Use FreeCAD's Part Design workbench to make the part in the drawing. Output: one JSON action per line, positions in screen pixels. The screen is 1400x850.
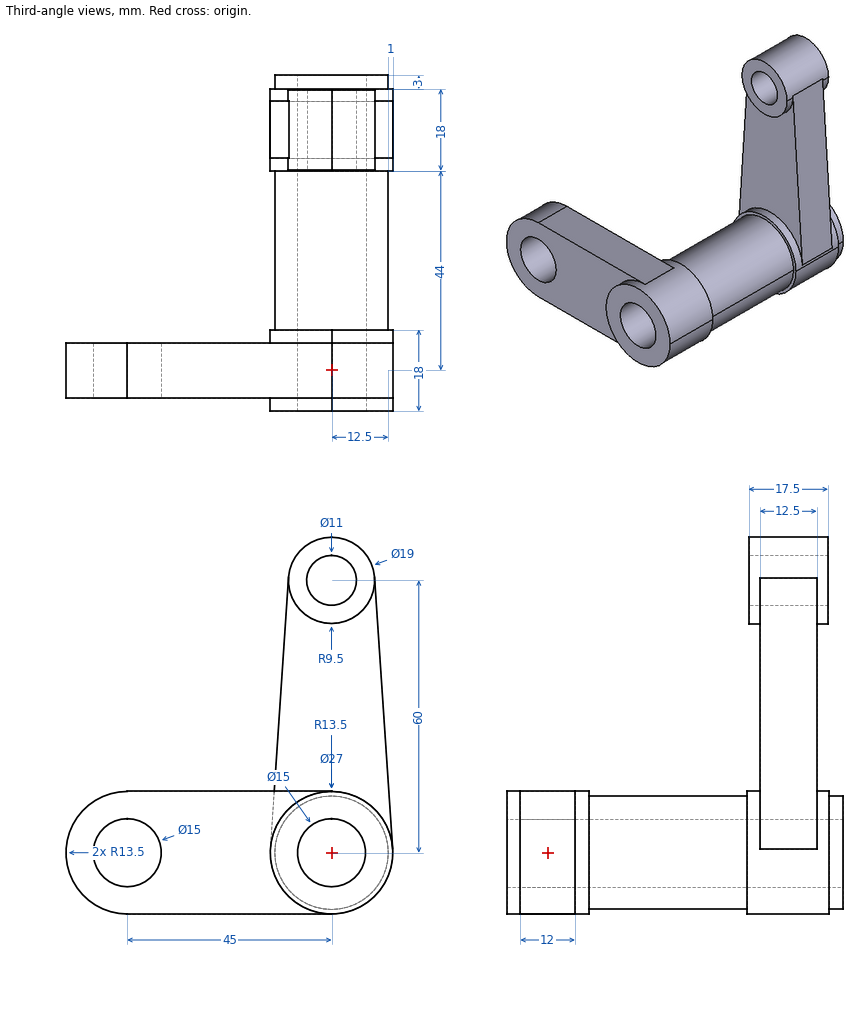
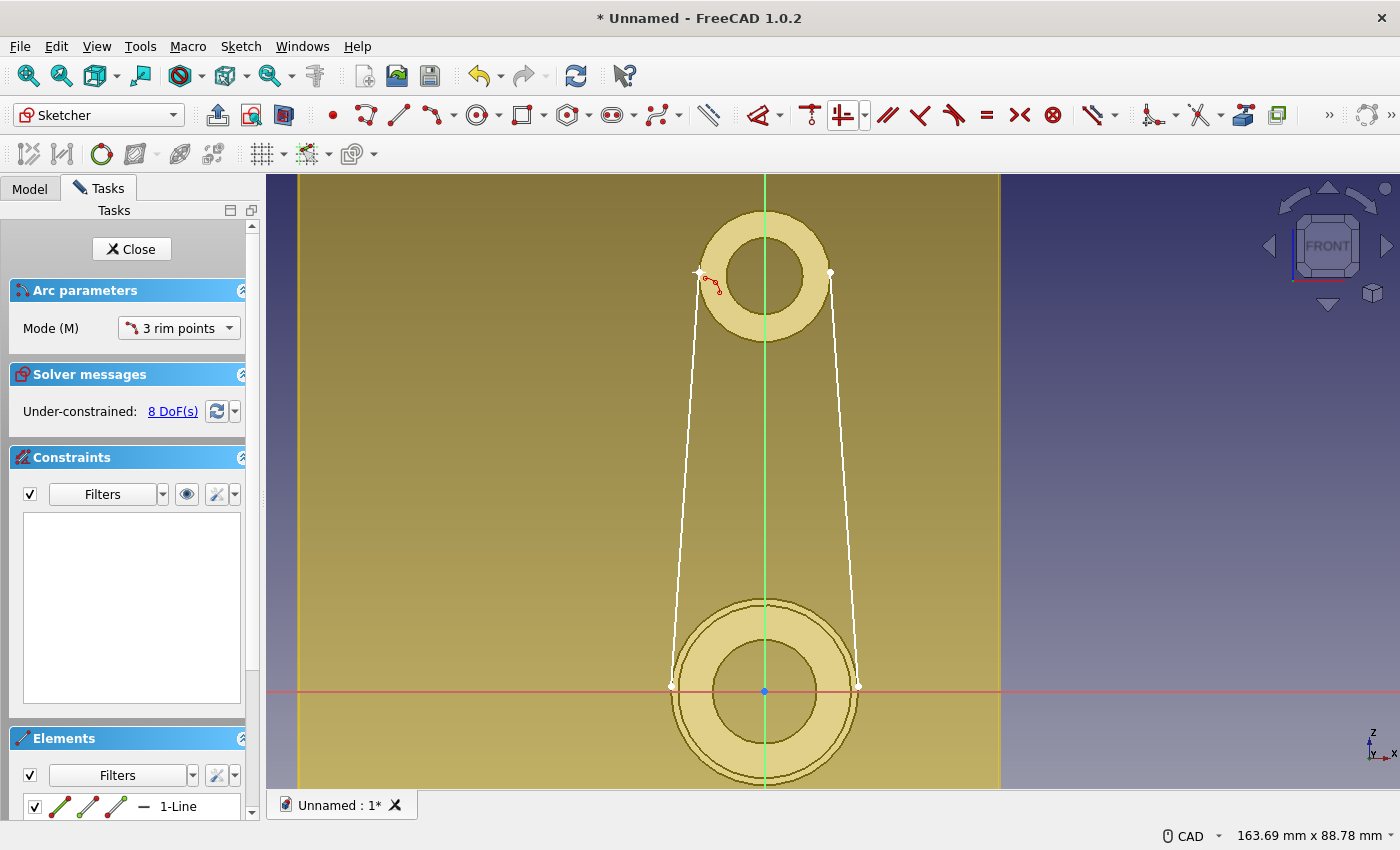
{"action": "scroll", "coordinate": [858, 686], "scroll_direction": "up", "scroll_amount": 5}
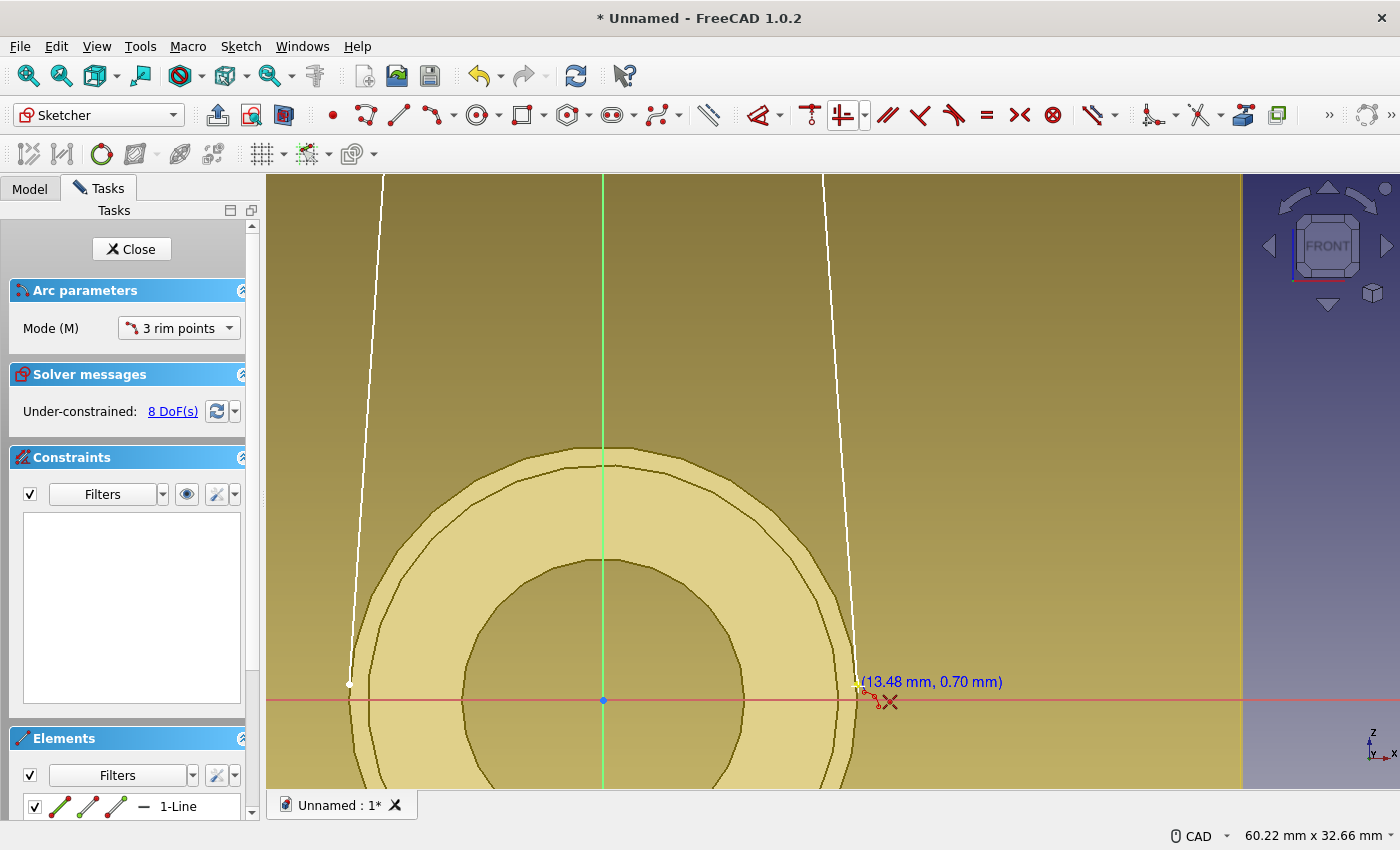
{"action": "left_click", "coordinate": [857, 685]}
{"action": "left_click", "coordinate": [349, 685]}
{"action": "left_click", "coordinate": [679, 458]}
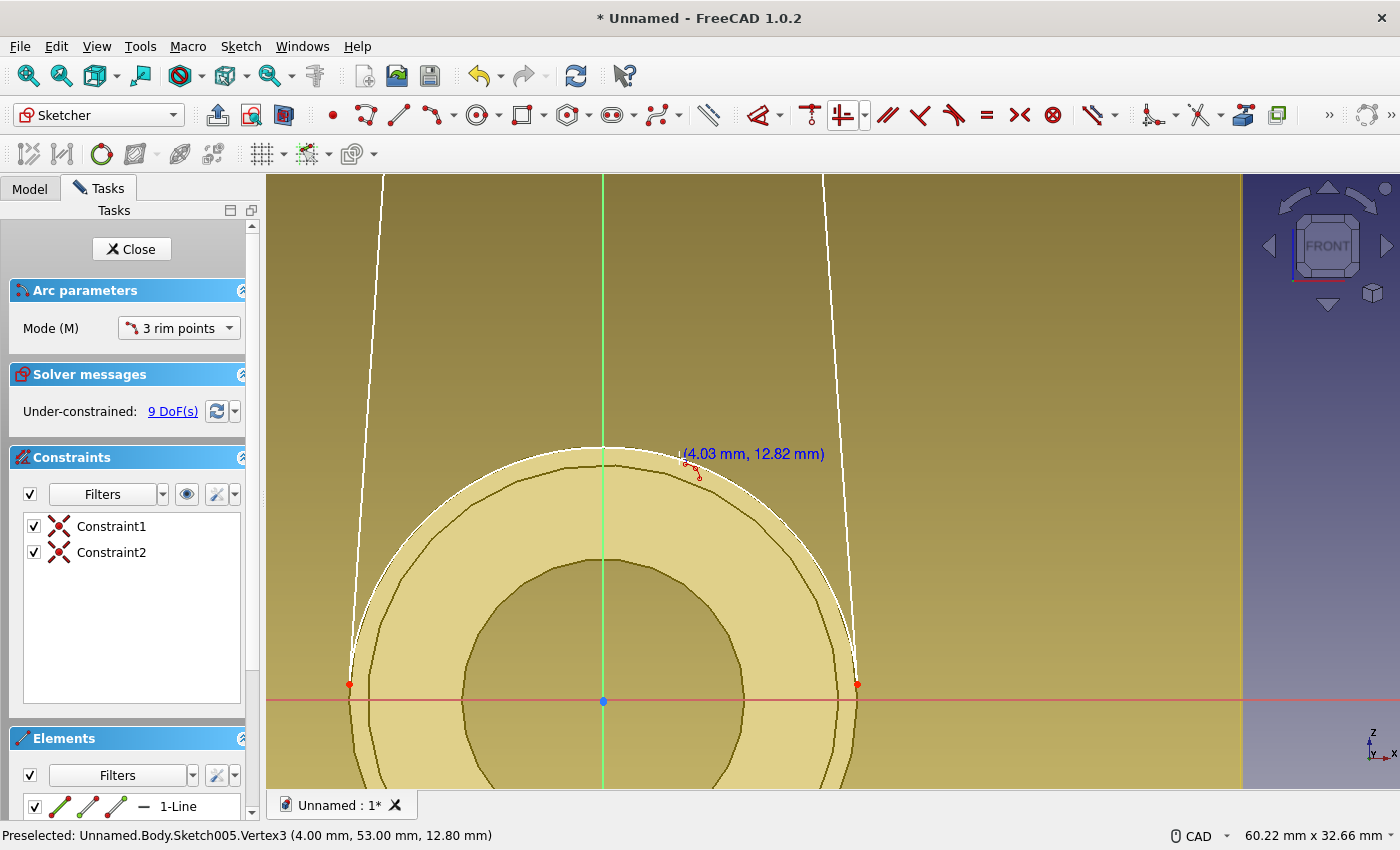
{"action": "scroll", "coordinate": [858, 686], "scroll_direction": "down", "scroll_amount": 5}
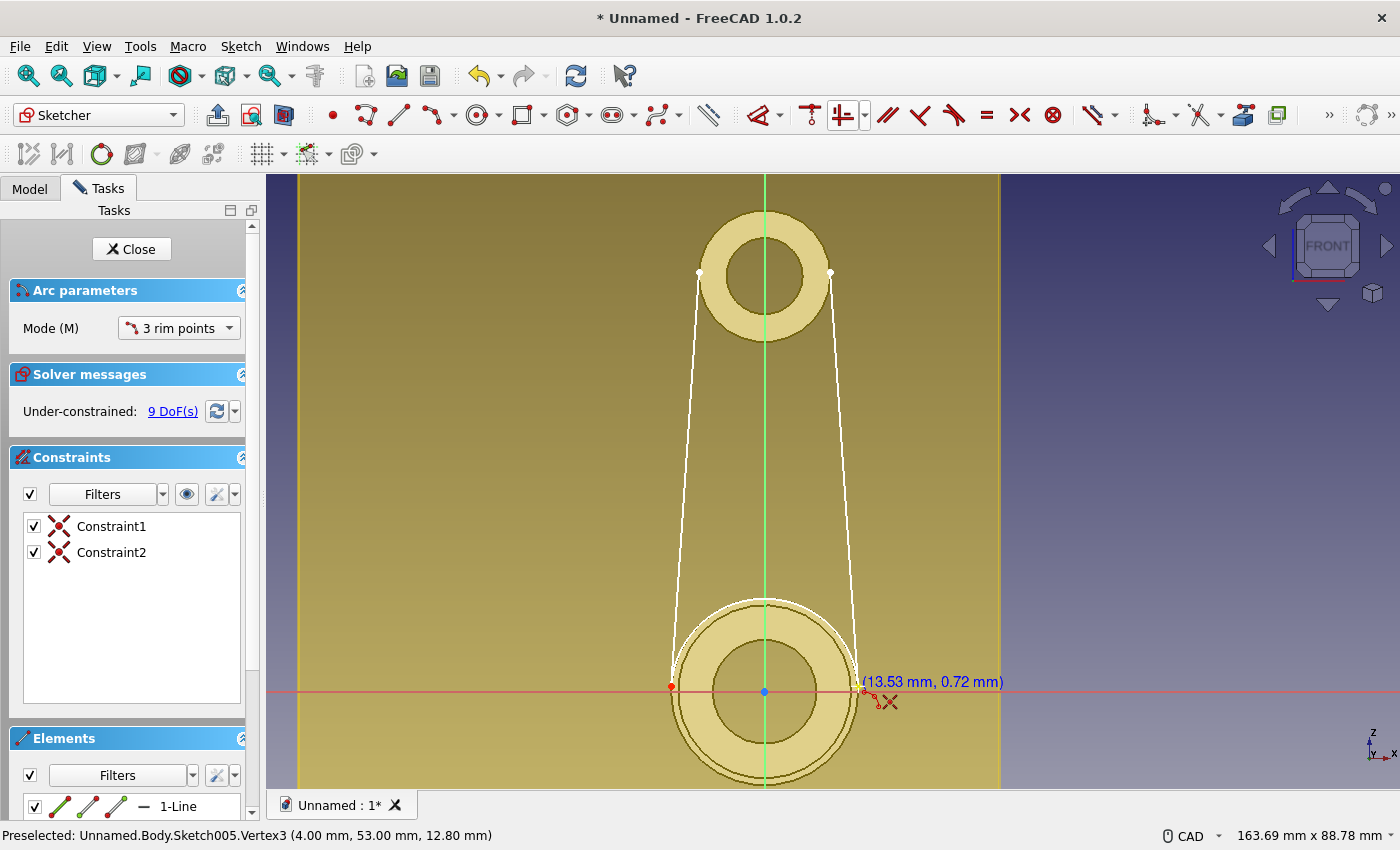
{"action": "left_click", "coordinate": [699, 273]}
{"action": "left_click", "coordinate": [830, 273]}
{"action": "left_click", "coordinate": [743, 339]}
{"action": "key", "text": "Escape"}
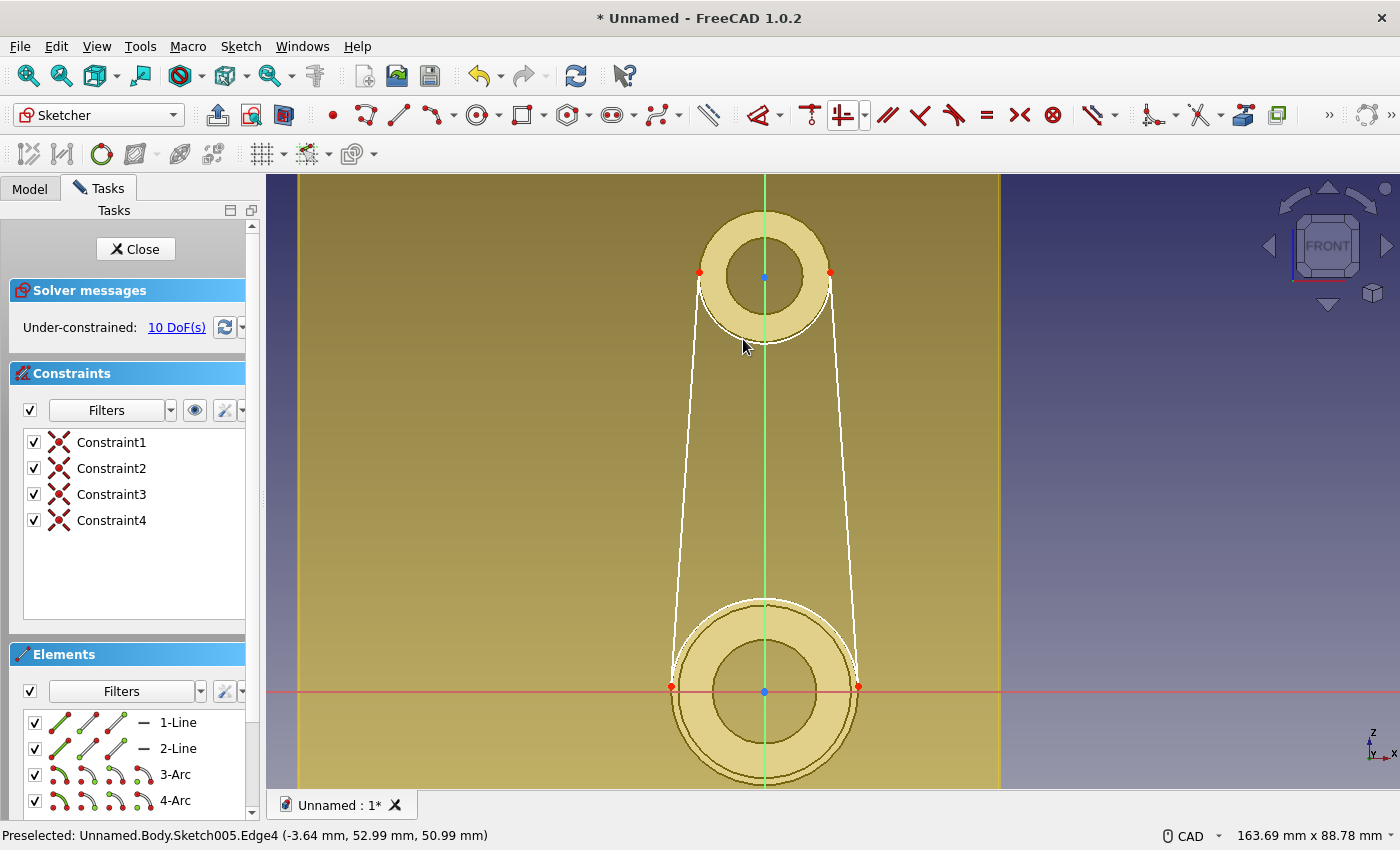
{"action": "left_click", "coordinate": [838, 397]}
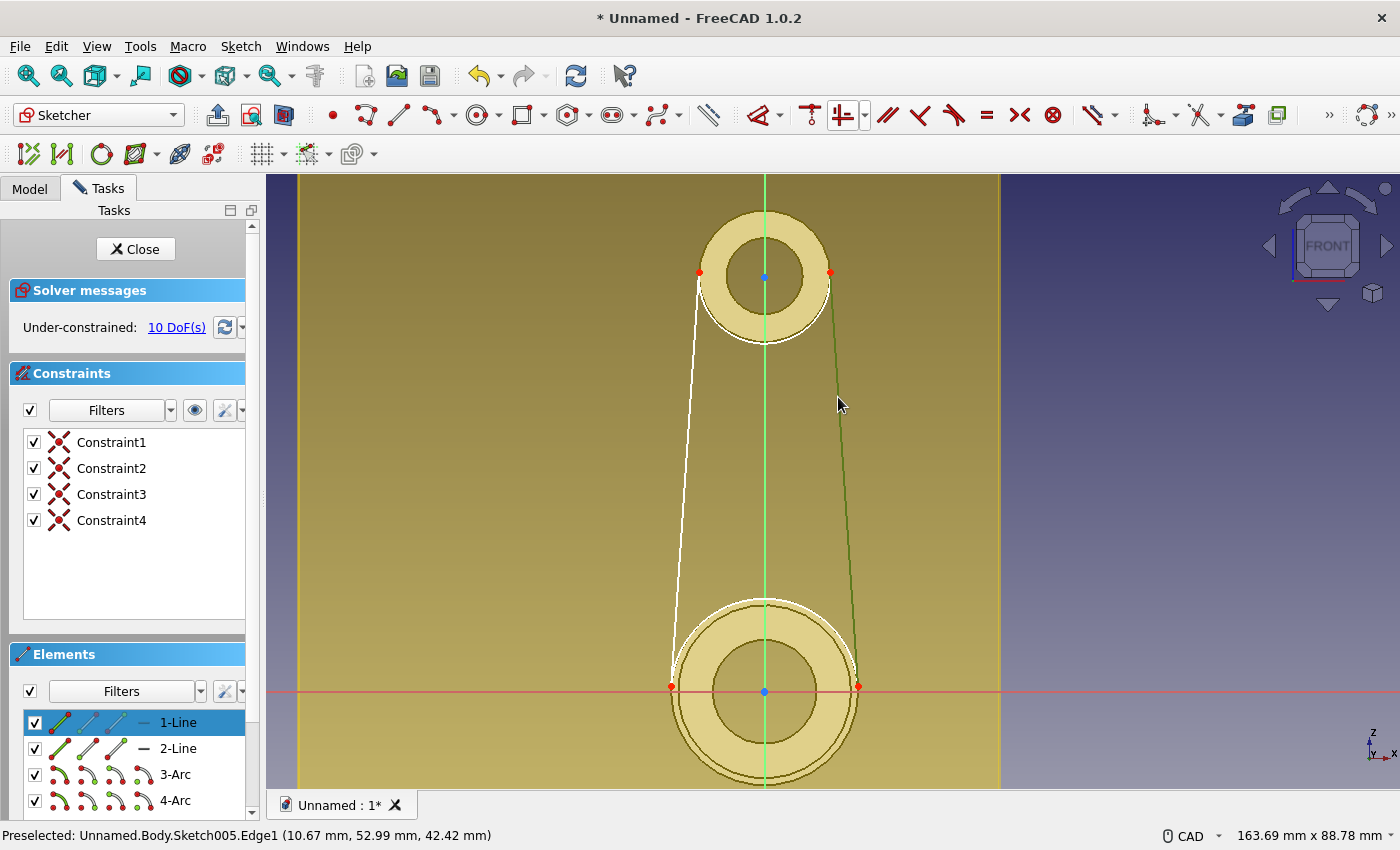
{"action": "left_click", "coordinate": [818, 615]}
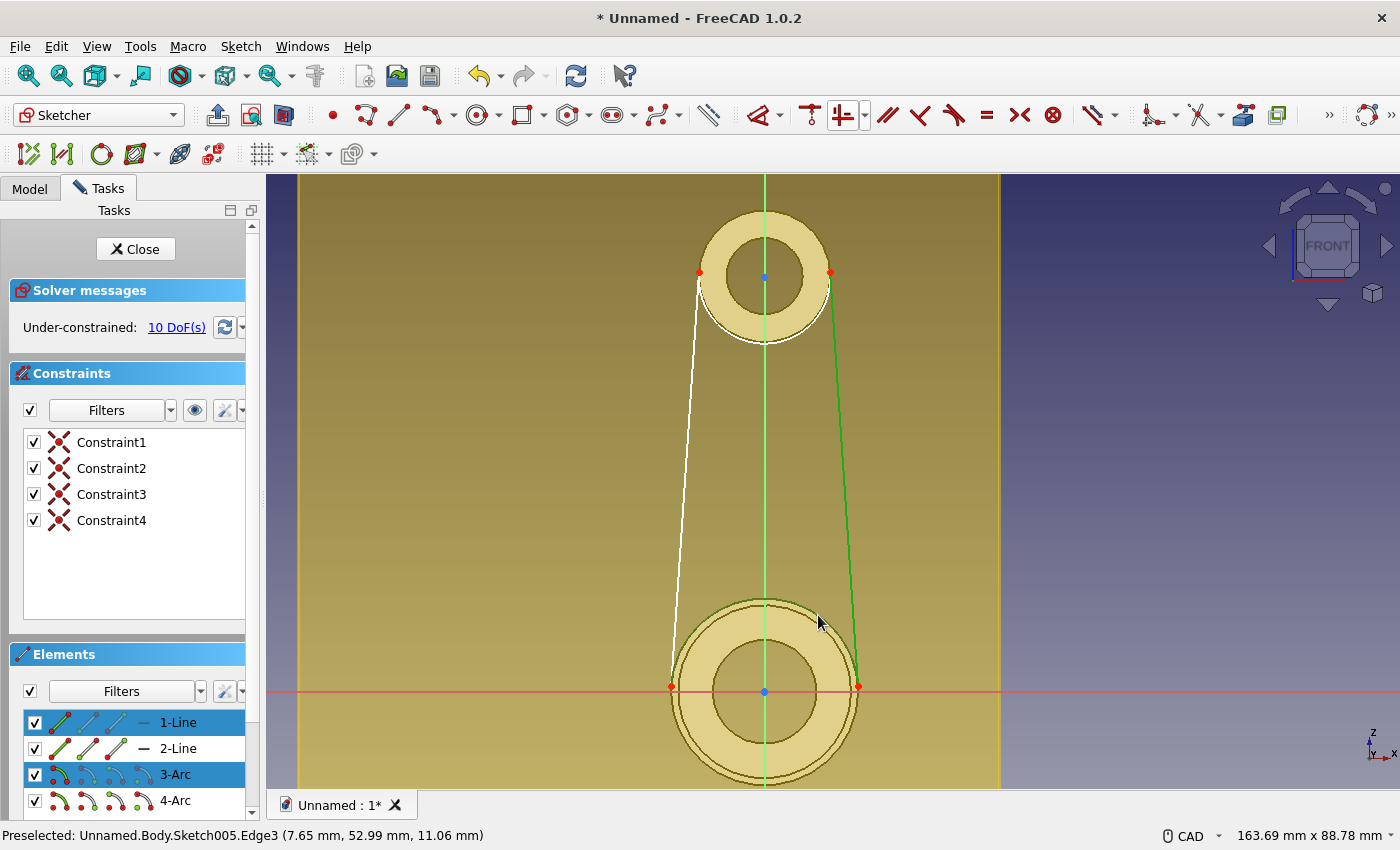
{"action": "key", "text": "t"}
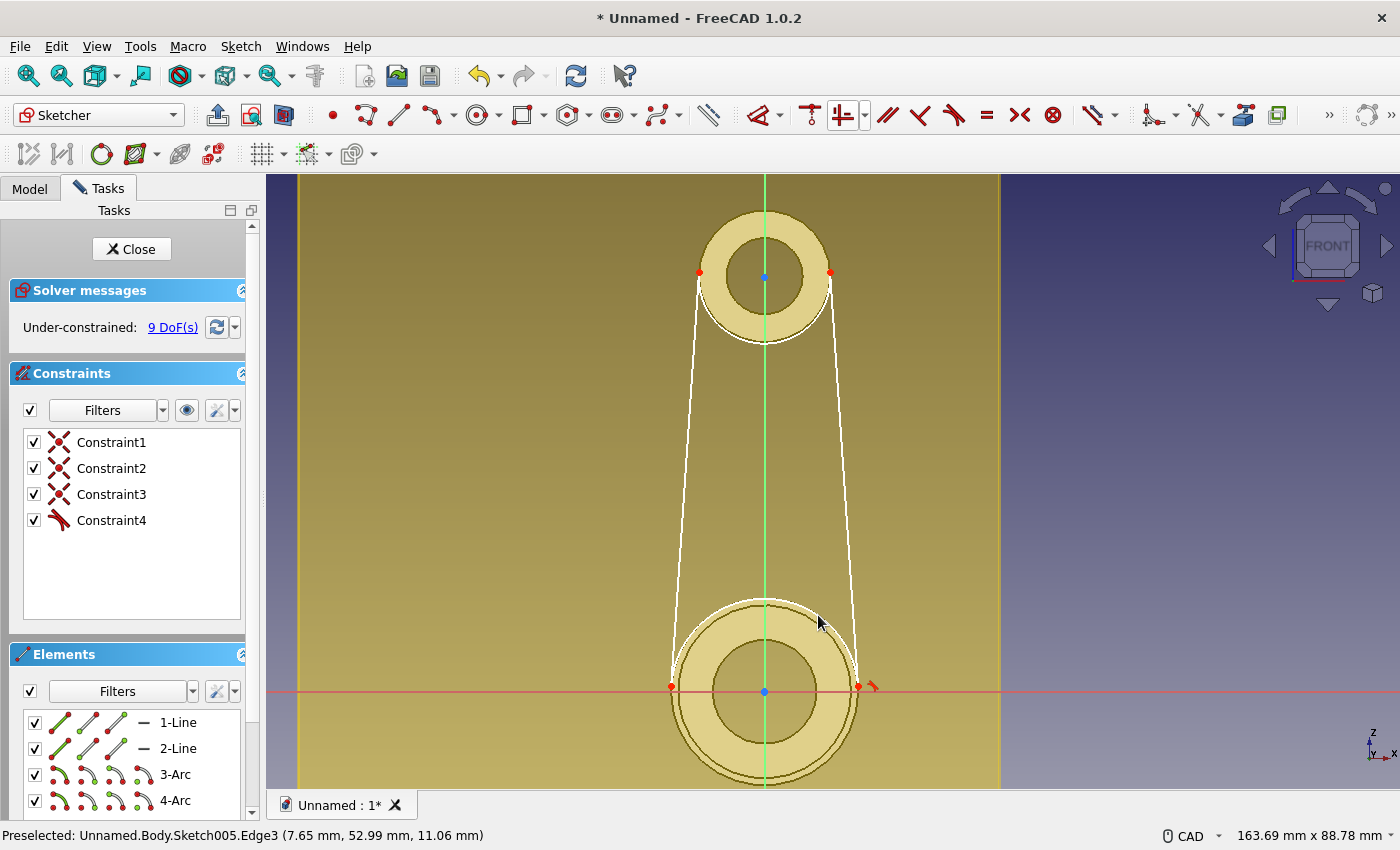
{"action": "left_click", "coordinate": [838, 397]}